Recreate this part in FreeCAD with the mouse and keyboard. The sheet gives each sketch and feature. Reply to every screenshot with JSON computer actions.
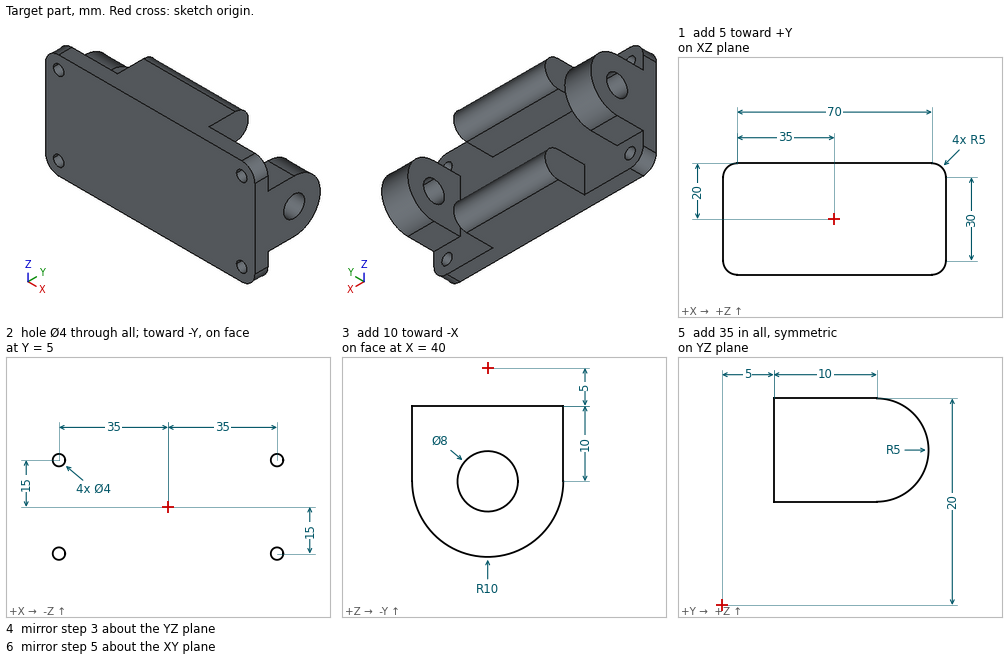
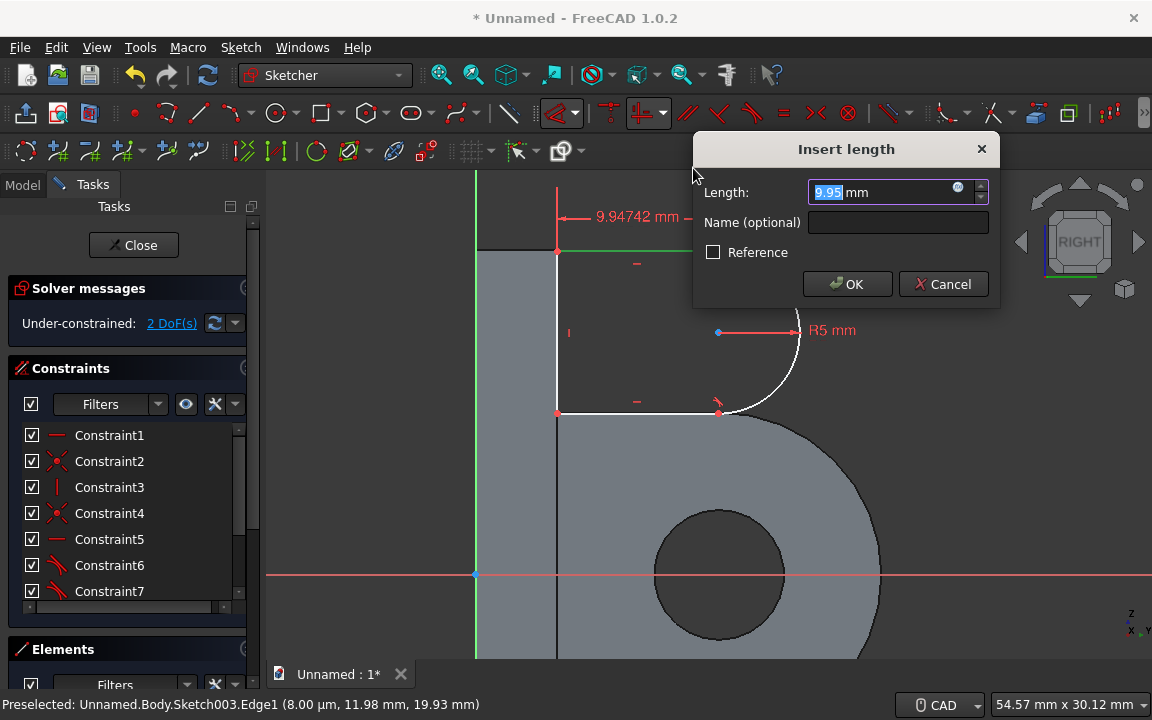
{"action": "type", "text": "10"}
{"action": "key", "text": "Return"}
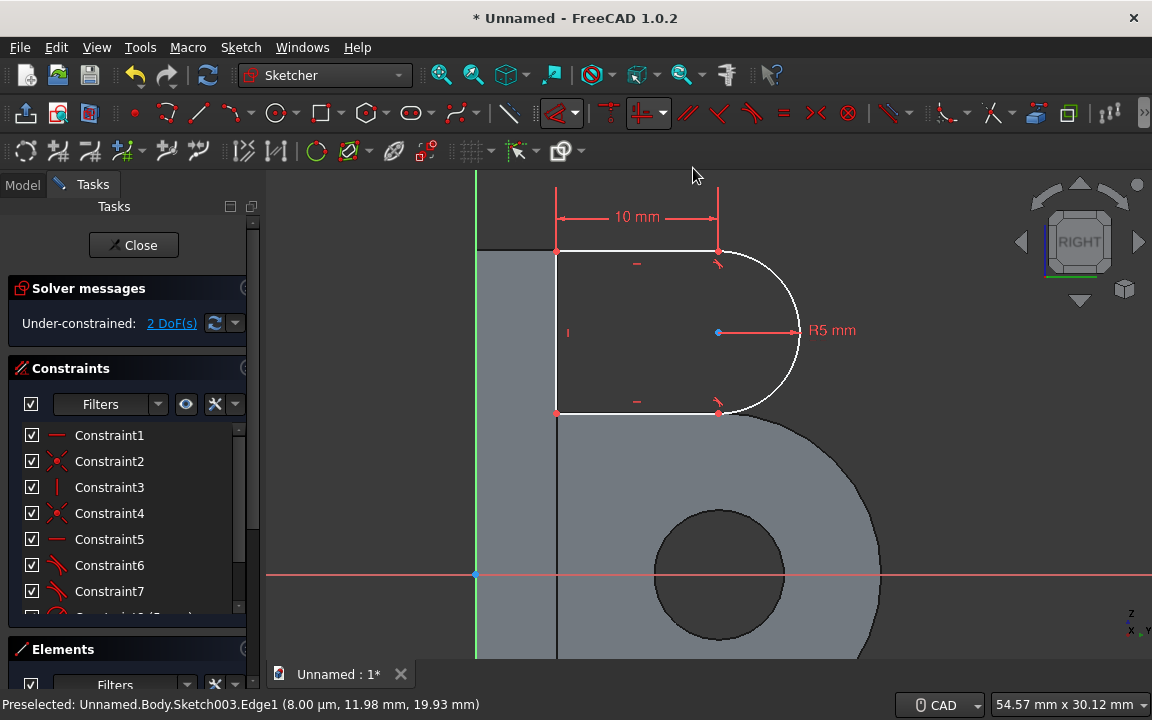
{"action": "left_click", "coordinate": [556, 251]}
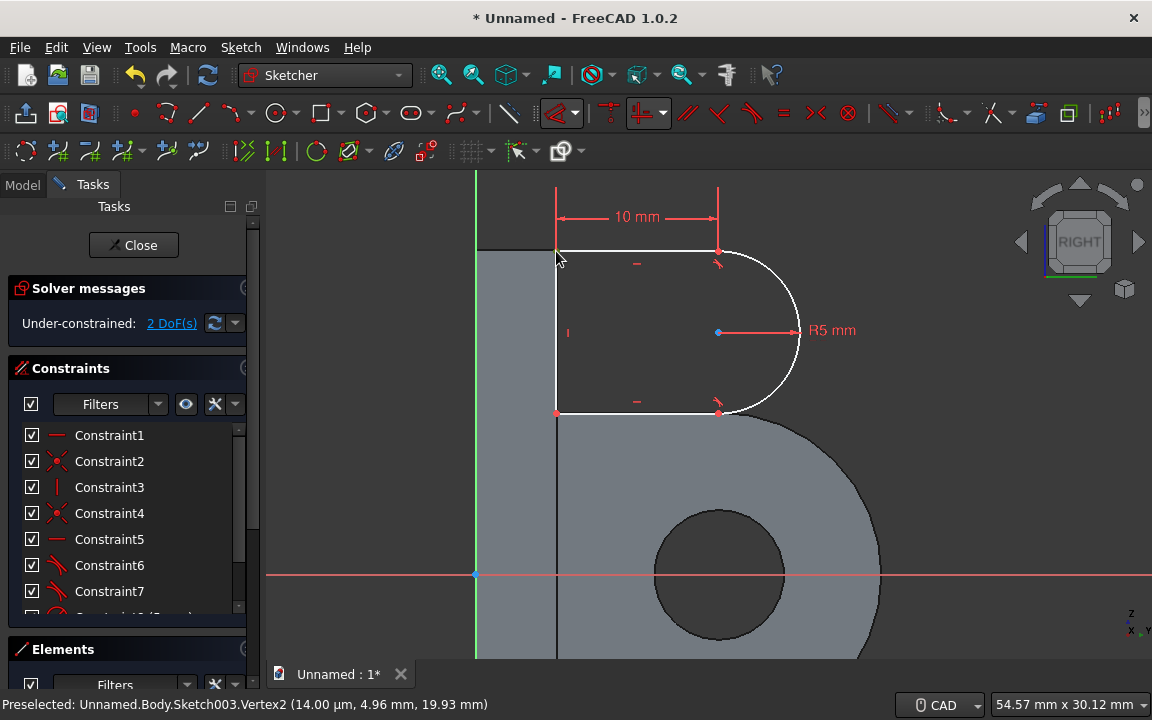
{"action": "key", "text": "l"}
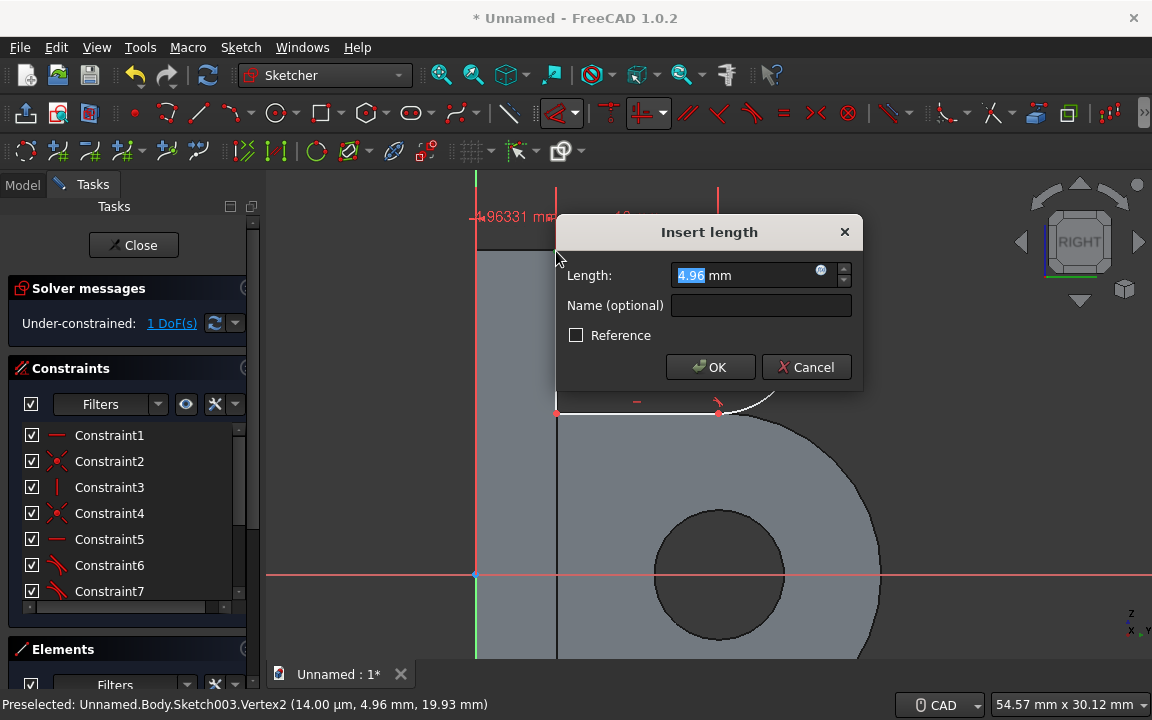
{"action": "type", "text": "5"}
{"action": "key", "text": "Return"}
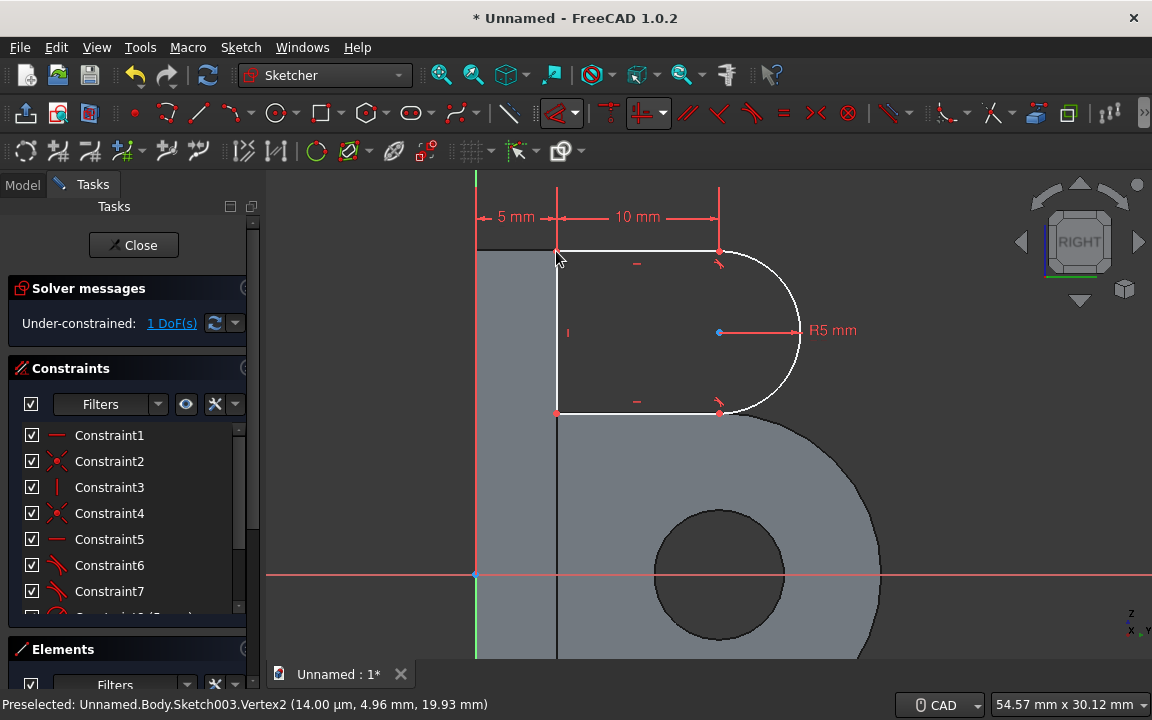
{"action": "left_click", "coordinate": [719, 251]}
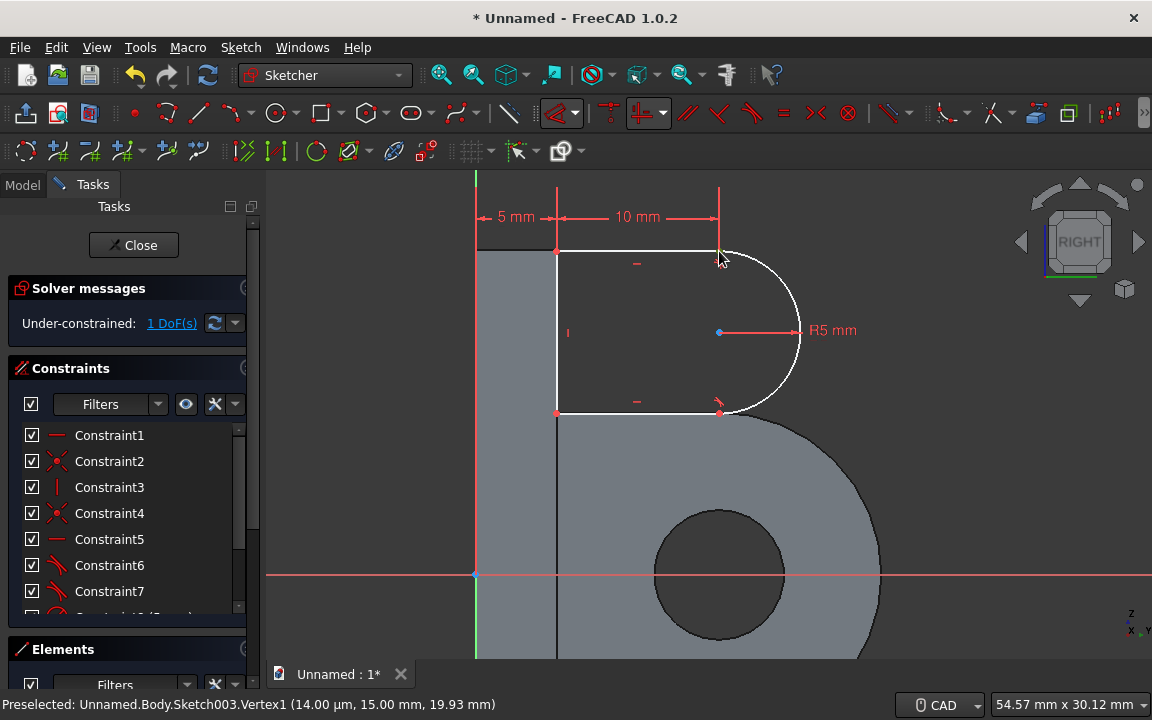
{"action": "key", "text": "i"}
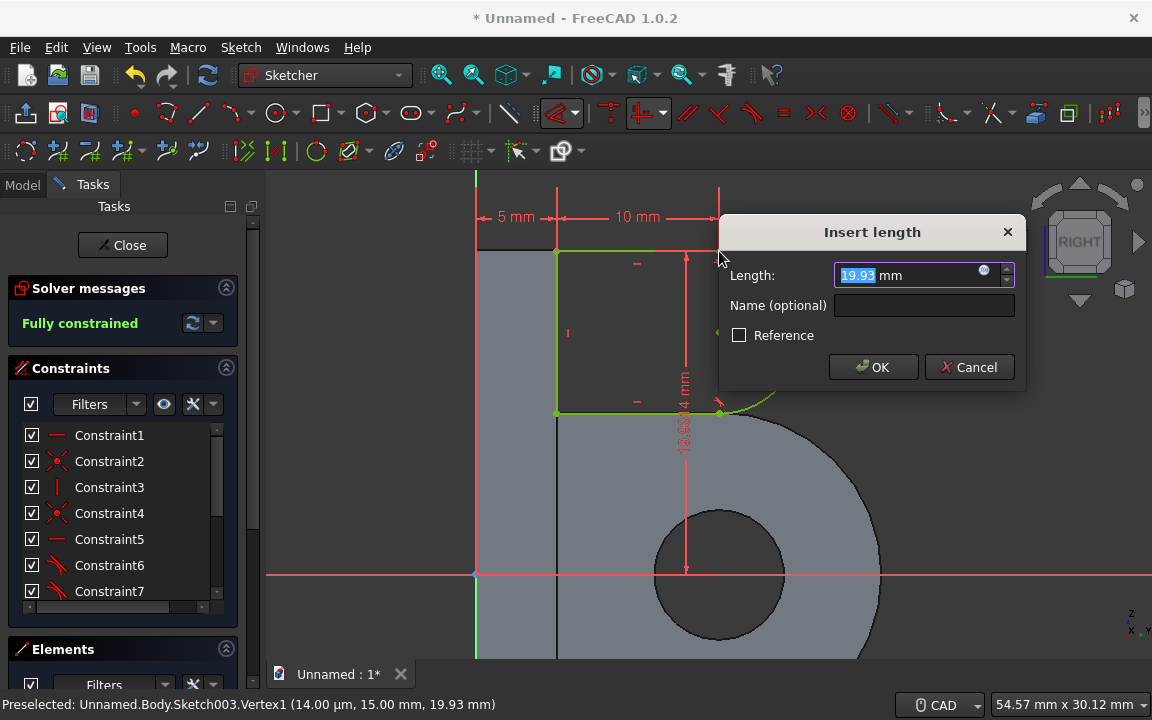
{"action": "type", "text": "20"}
{"action": "key", "text": "Return"}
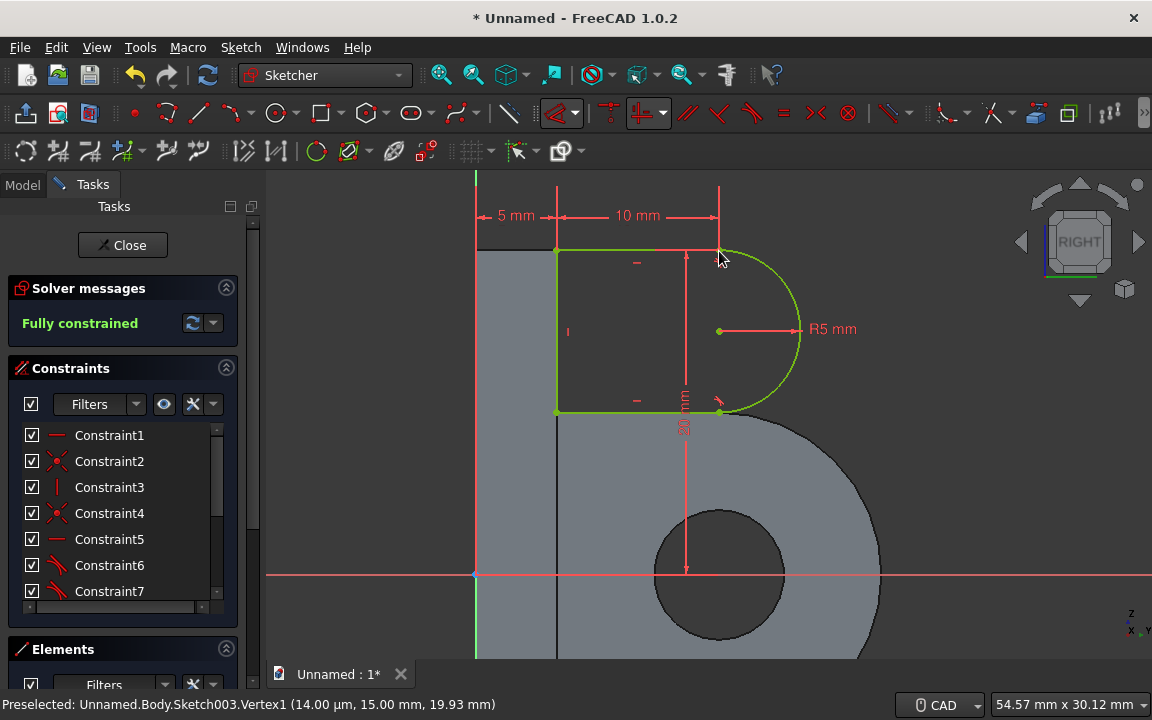
{"action": "left_click", "coordinate": [123, 245]}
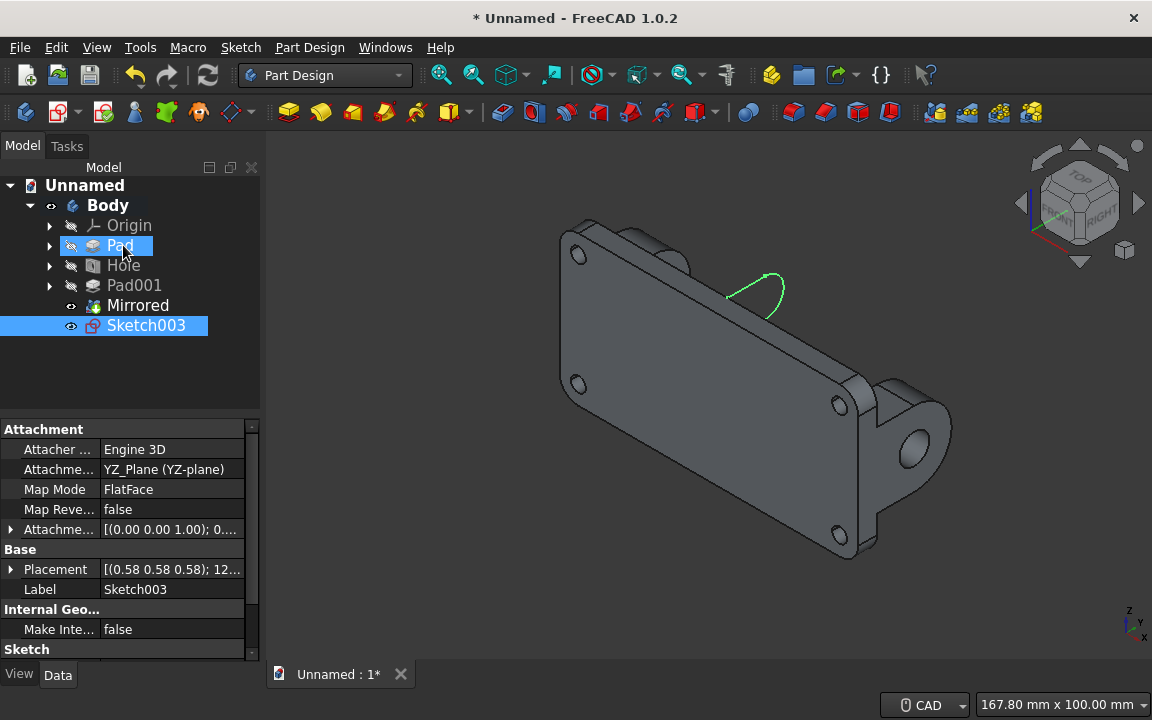
{"action": "left_click", "coordinate": [290, 112]}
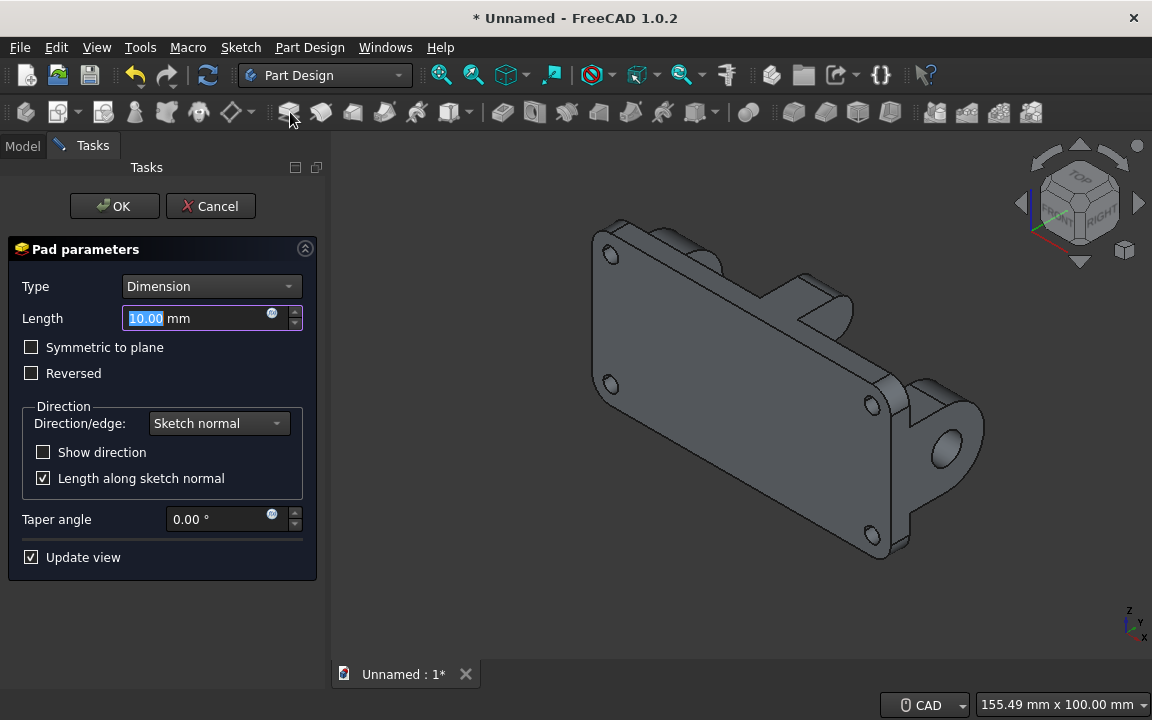
{"action": "type", "text": "35"}
{"action": "key", "text": "Tab"}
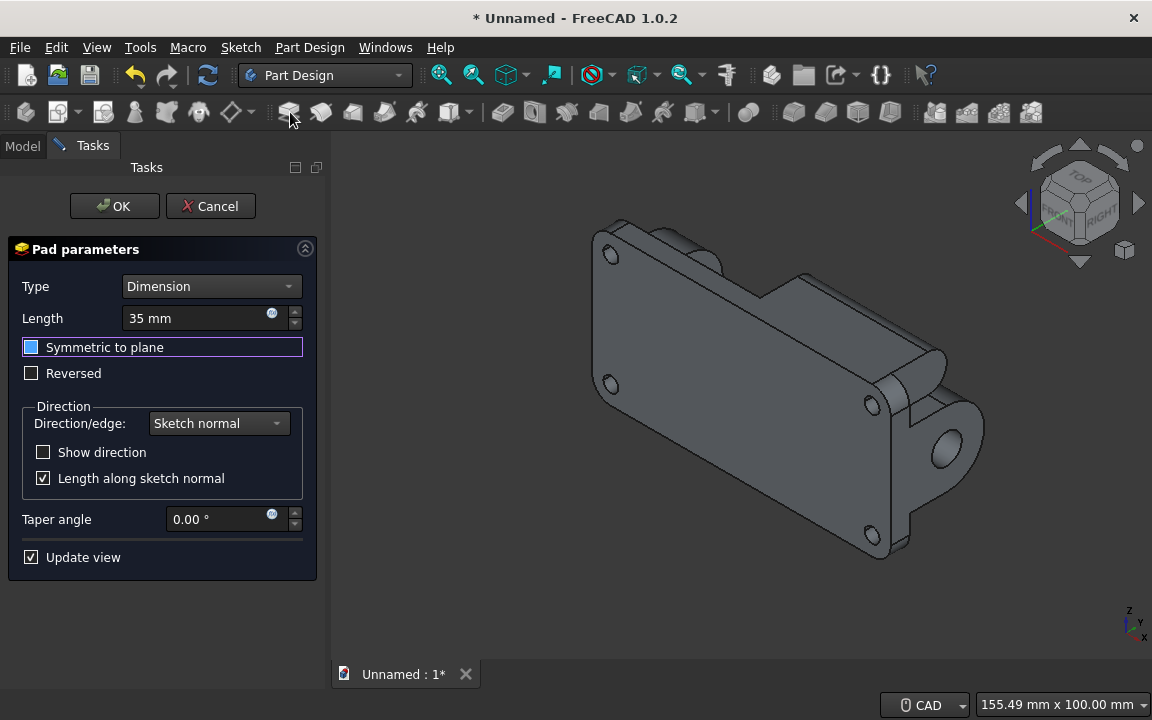
{"action": "left_click", "coordinate": [30, 347]}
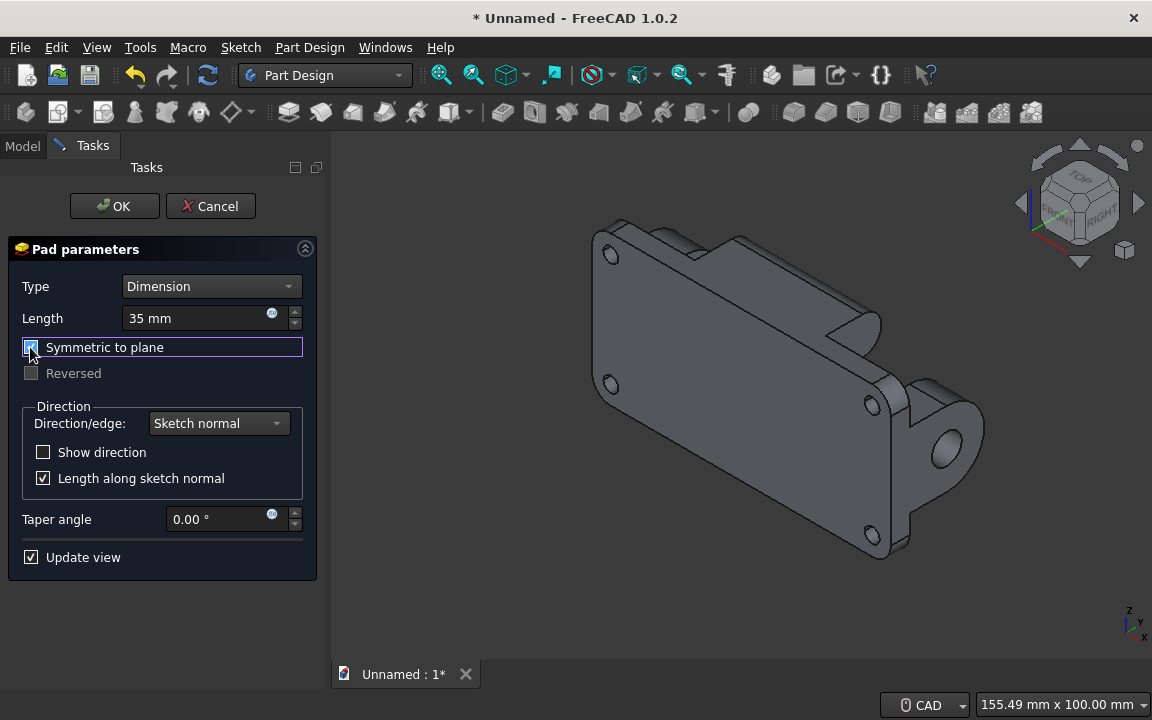
{"action": "left_click", "coordinate": [115, 206]}